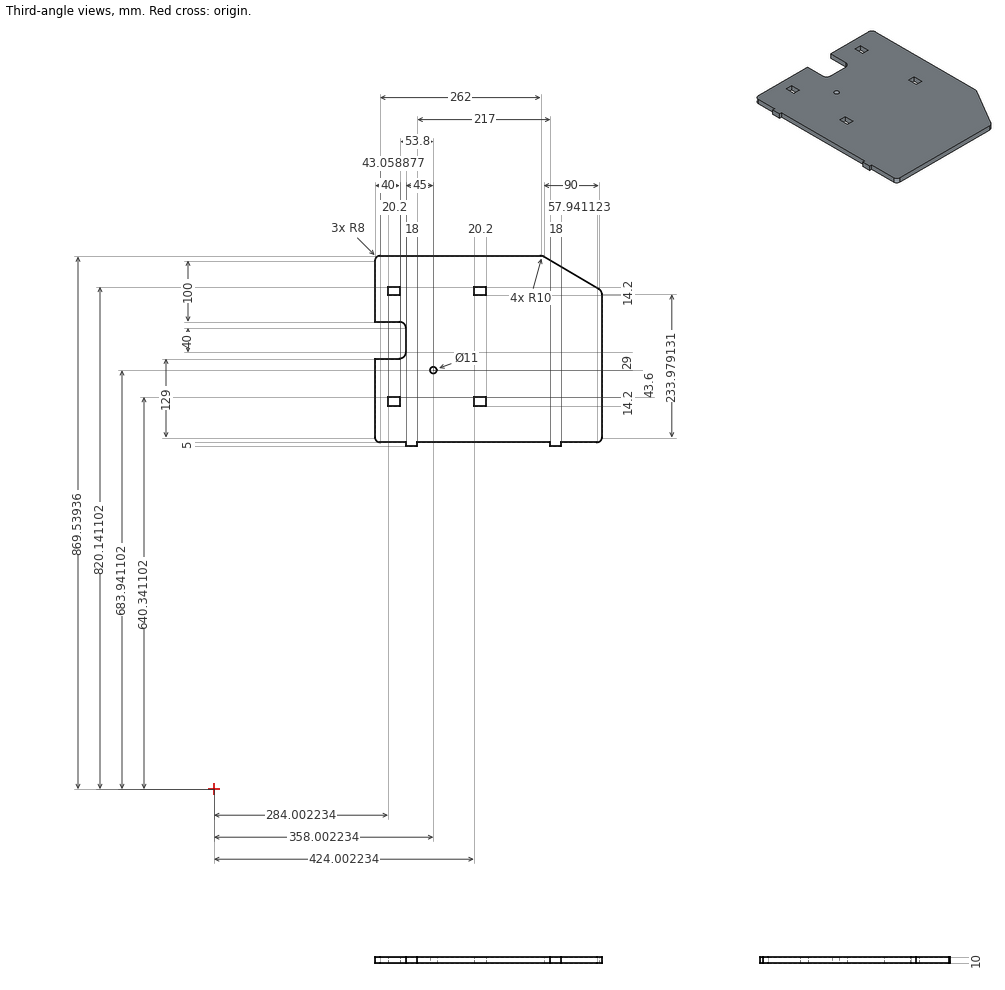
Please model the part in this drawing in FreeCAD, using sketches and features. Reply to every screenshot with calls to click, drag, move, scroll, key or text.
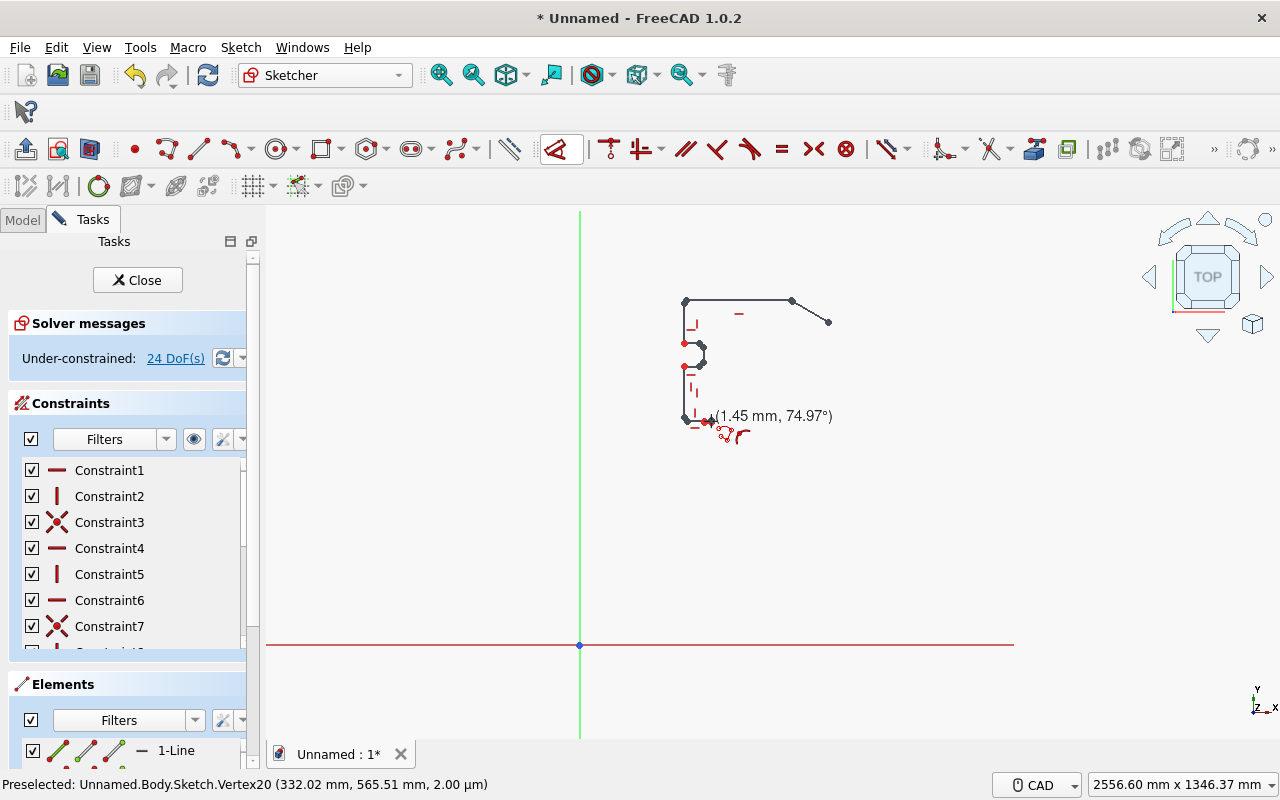
click(797, 421)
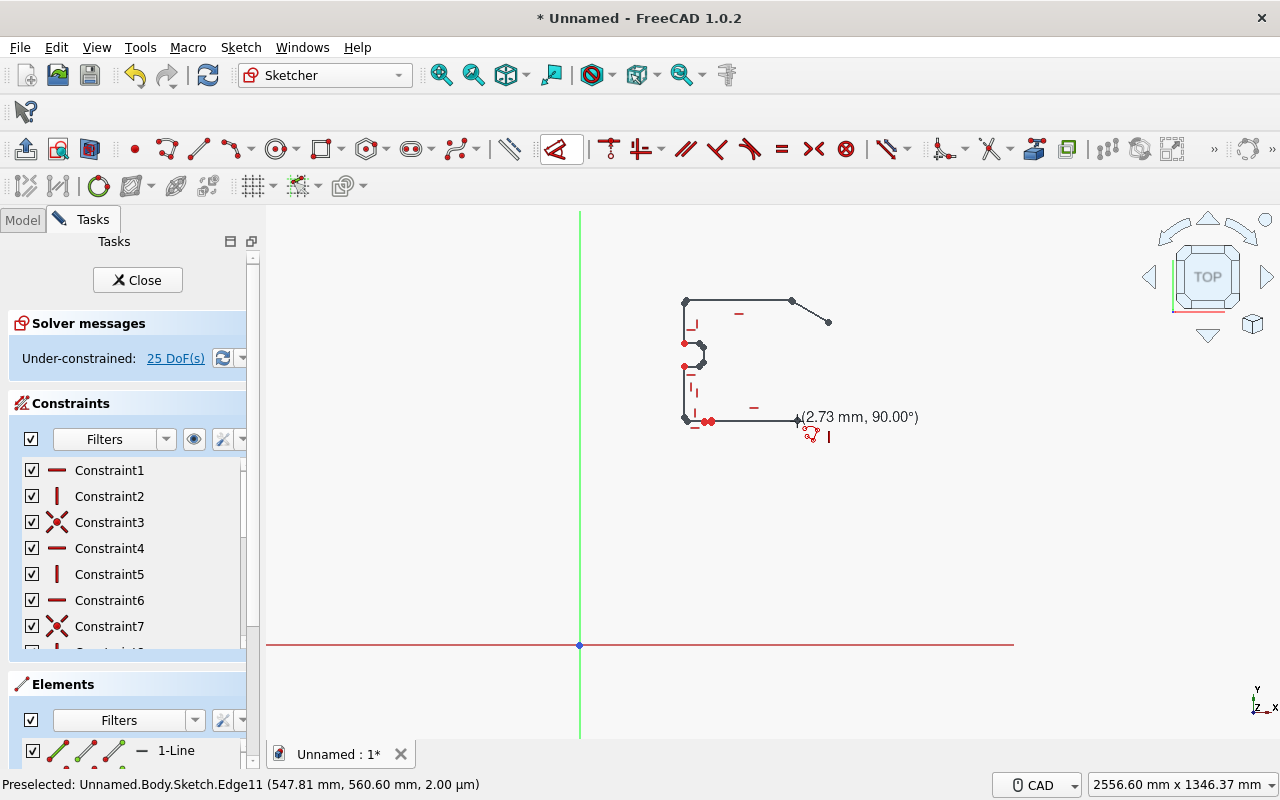
scroll(797, 423, up, 11)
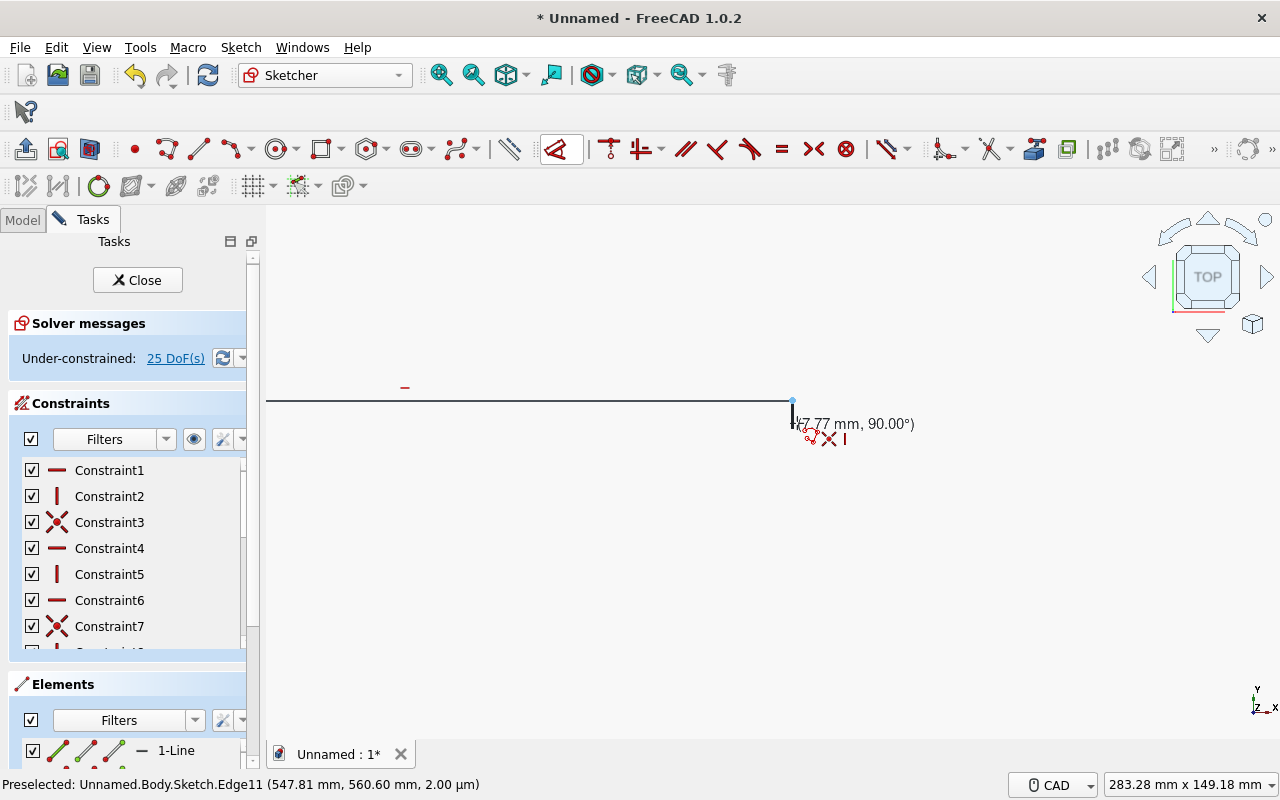
click(793, 418)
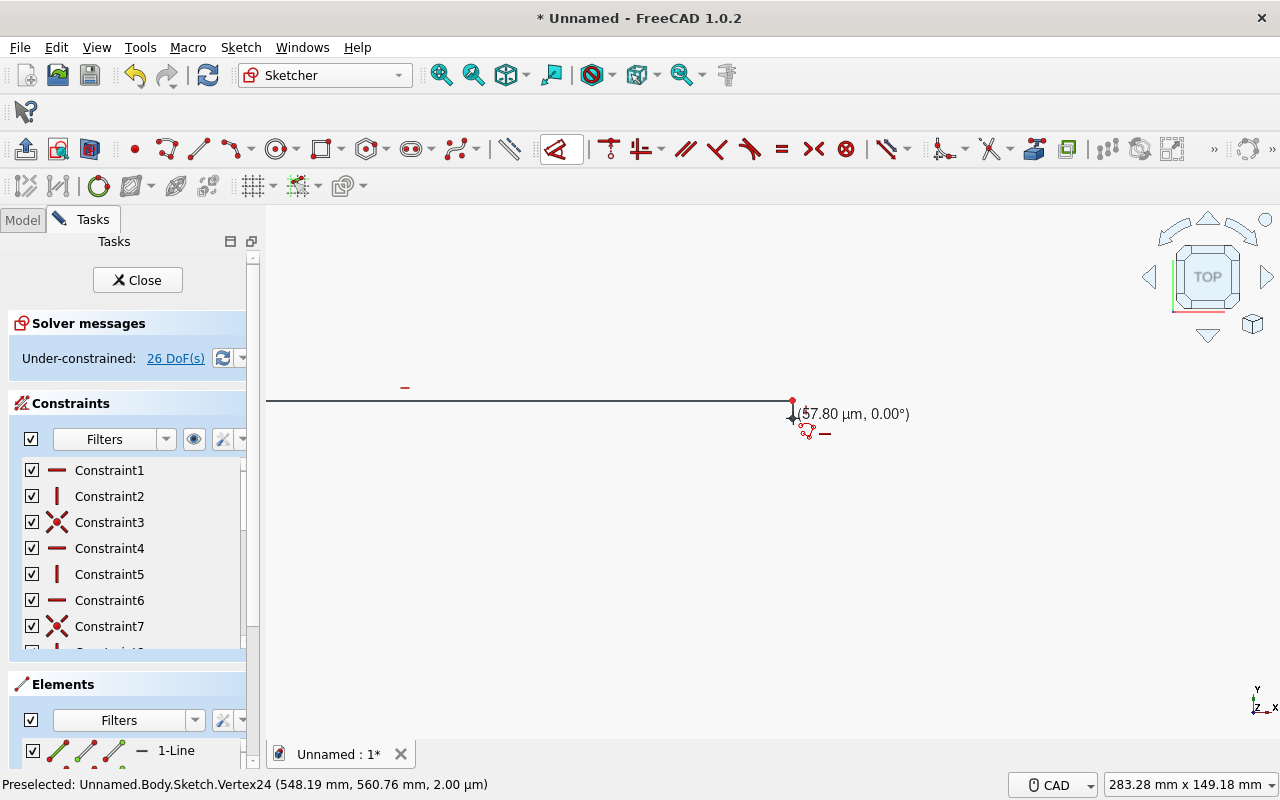
scroll(797, 423, down, 11)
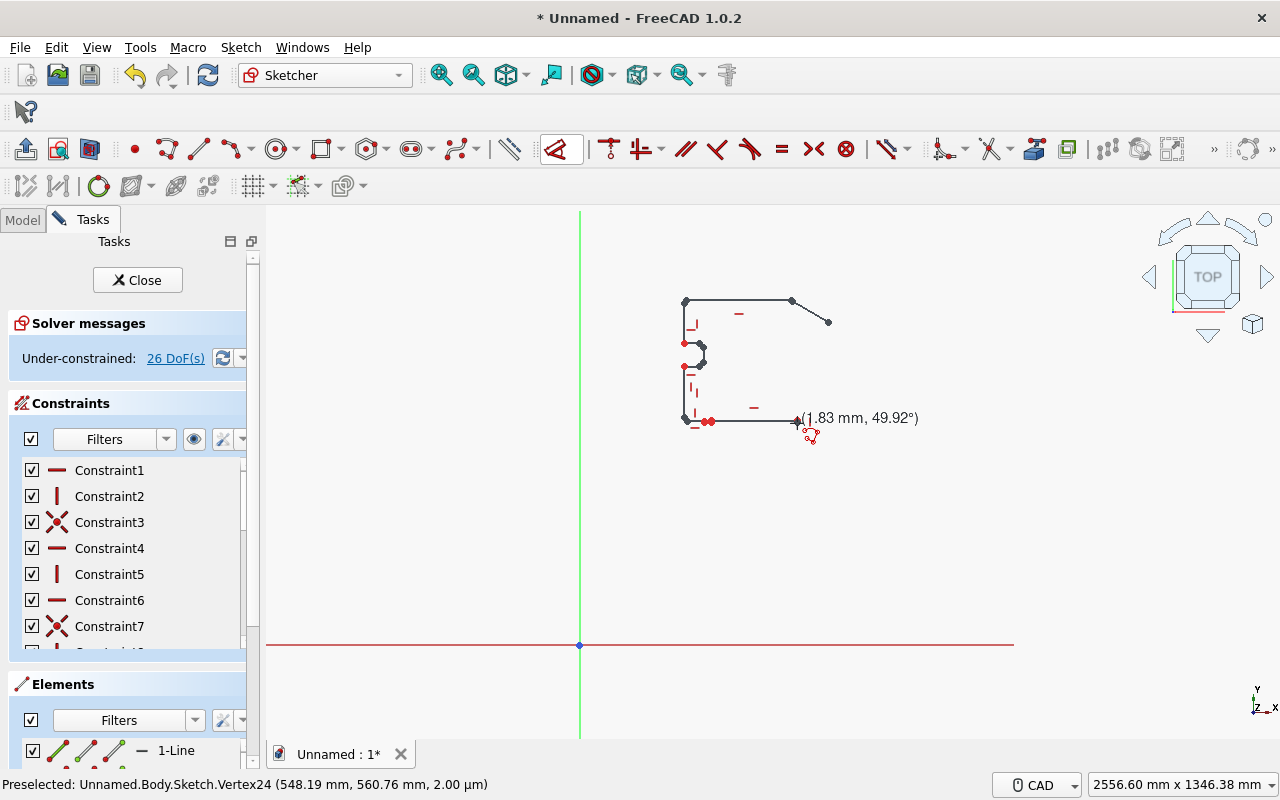
scroll(805, 423, up, 4)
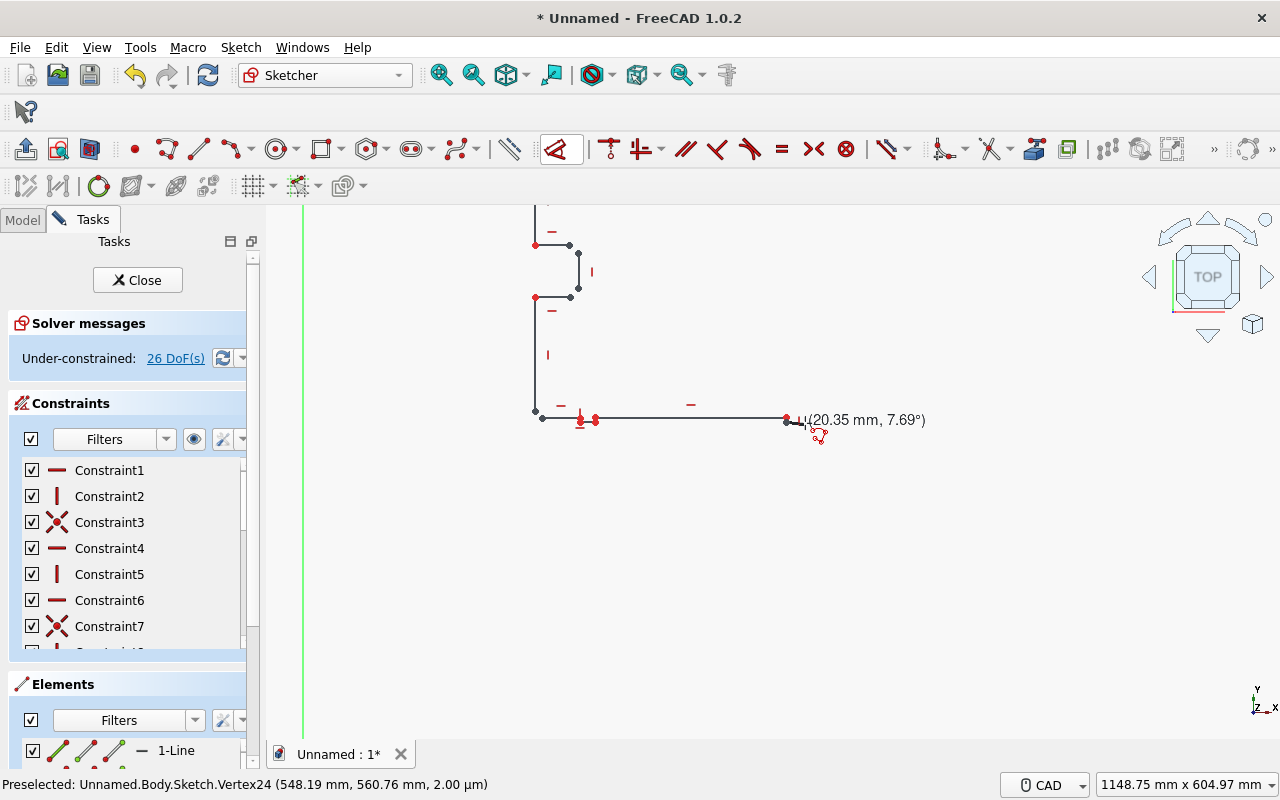
click(803, 422)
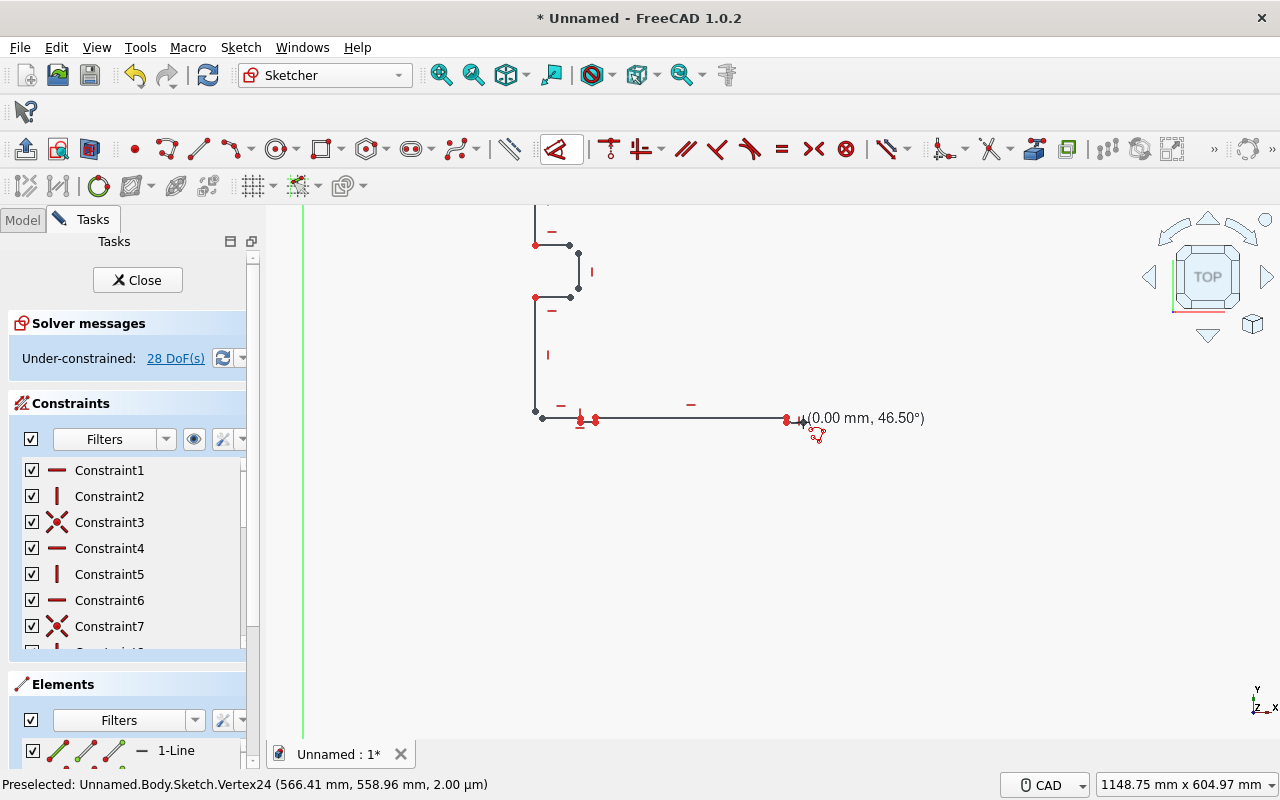
scroll(803, 418, up, 7)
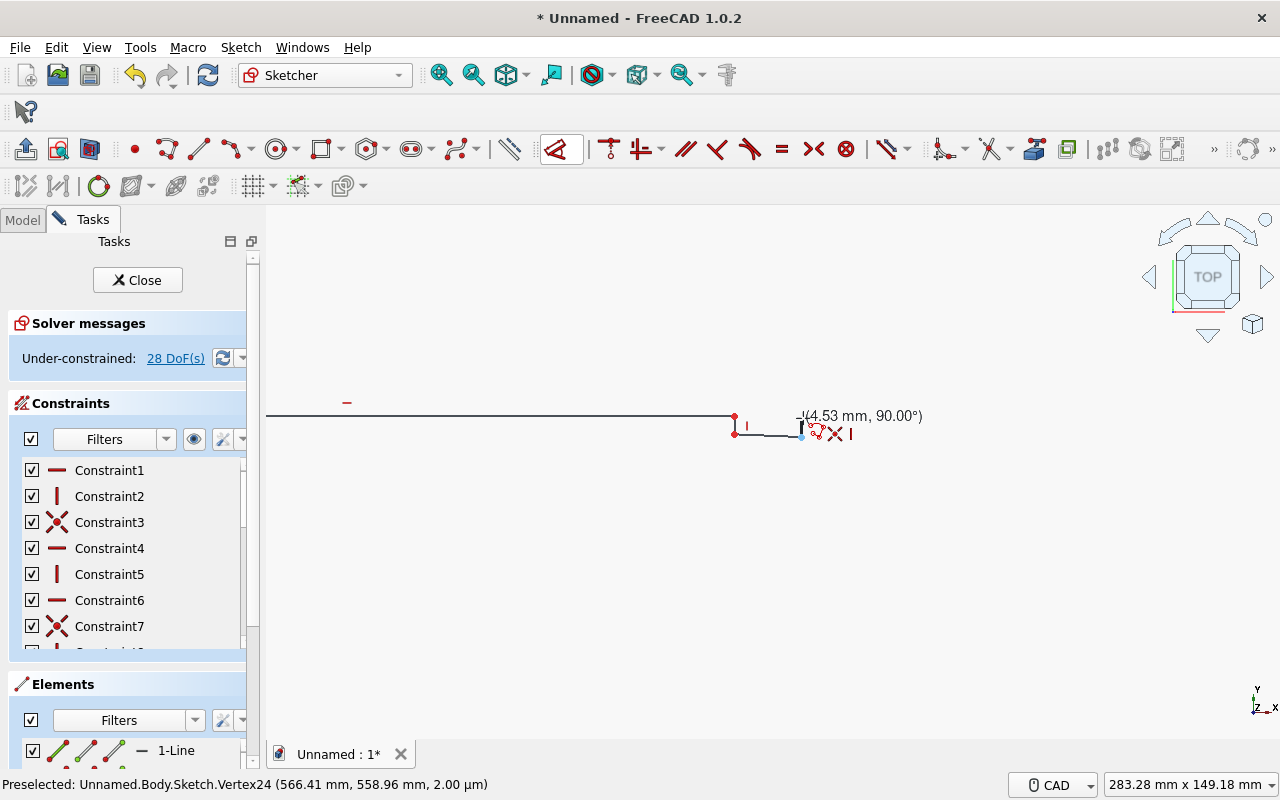
click(801, 416)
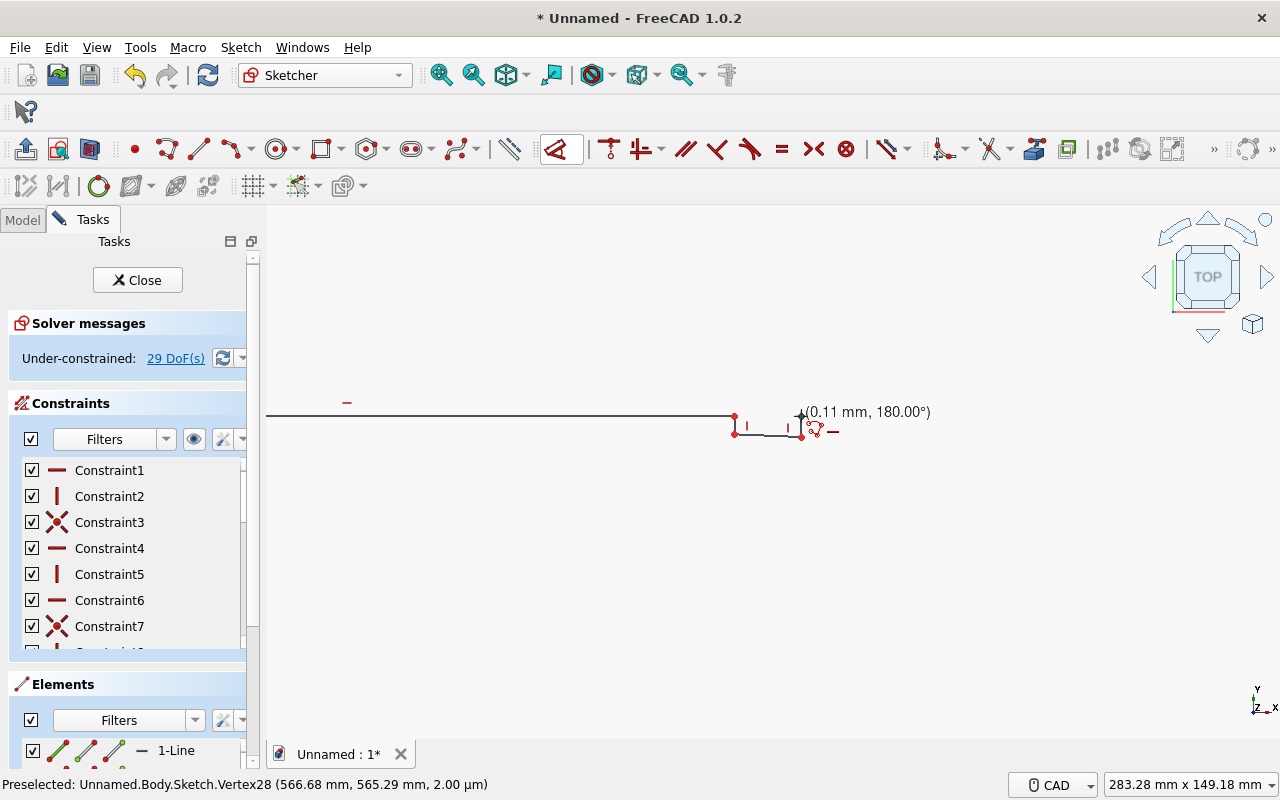
scroll(804, 421, down, 11)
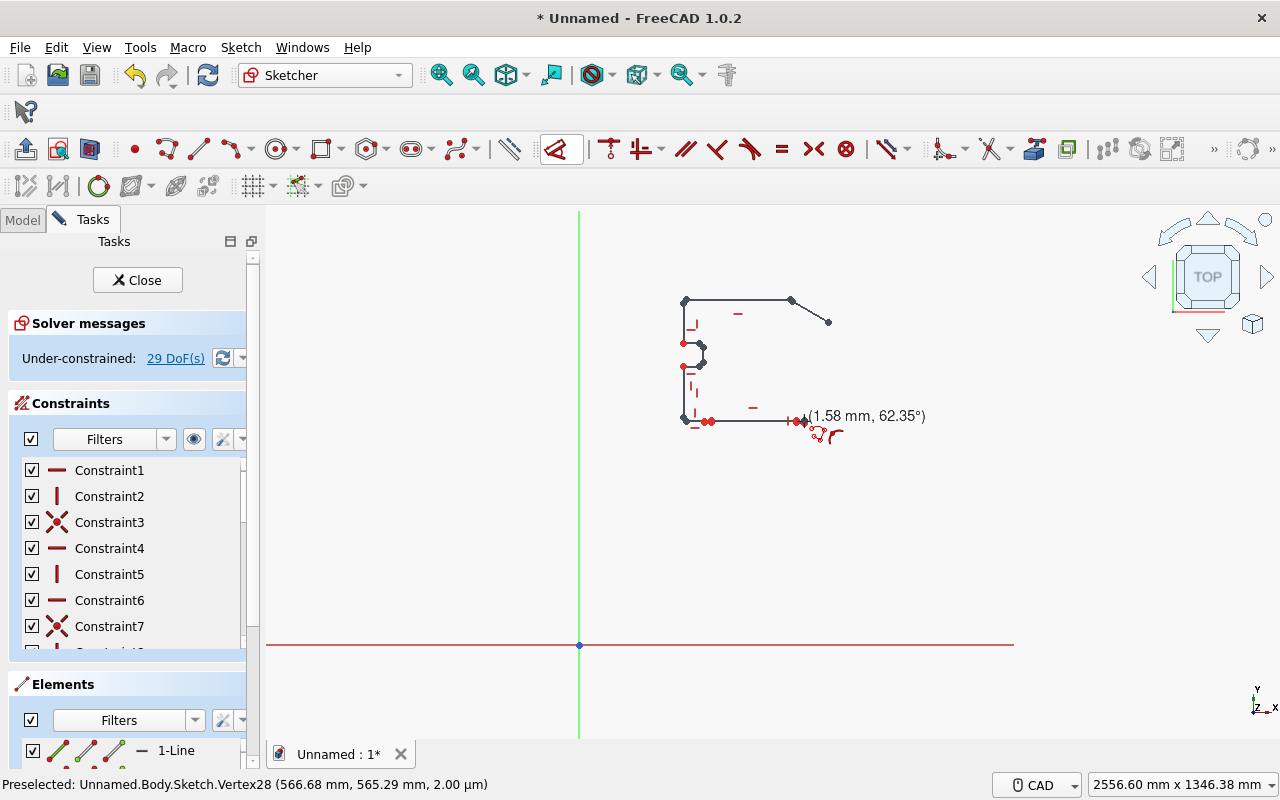
click(827, 421)
right_click(827, 421)